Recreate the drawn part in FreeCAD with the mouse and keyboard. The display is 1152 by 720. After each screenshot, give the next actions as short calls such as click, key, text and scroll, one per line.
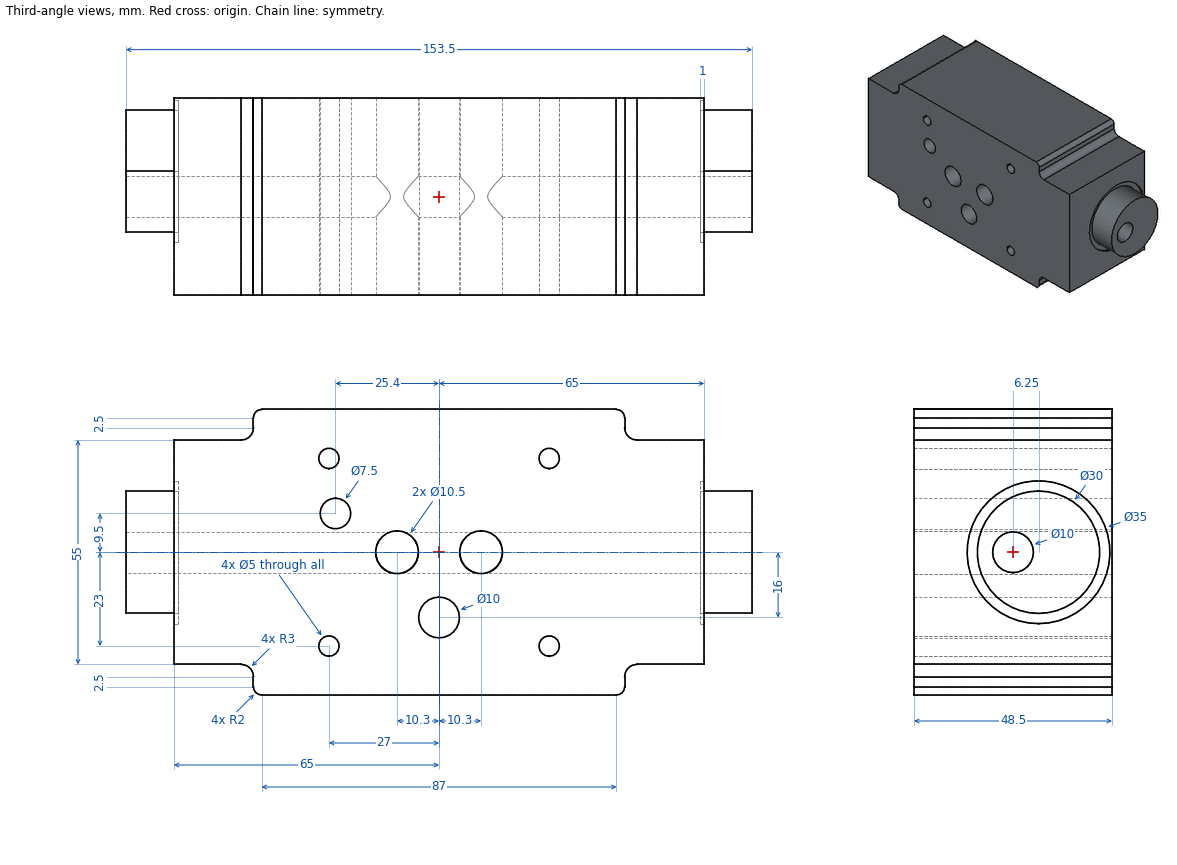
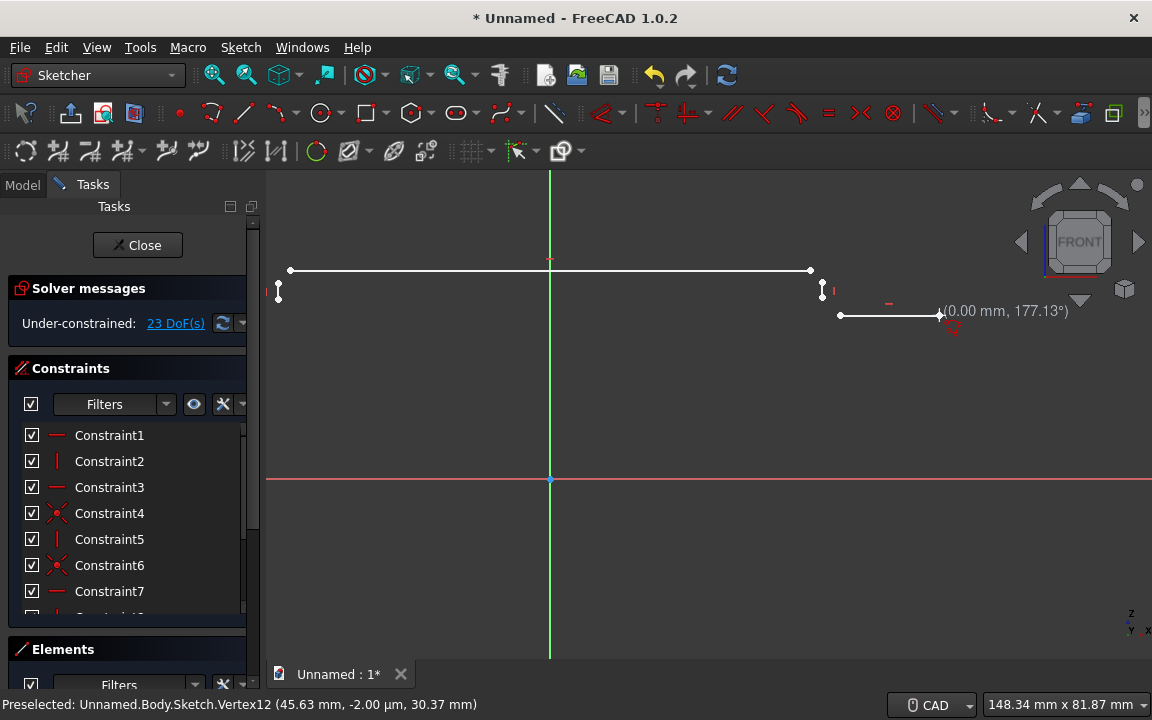
scroll(824, 283, down, 2)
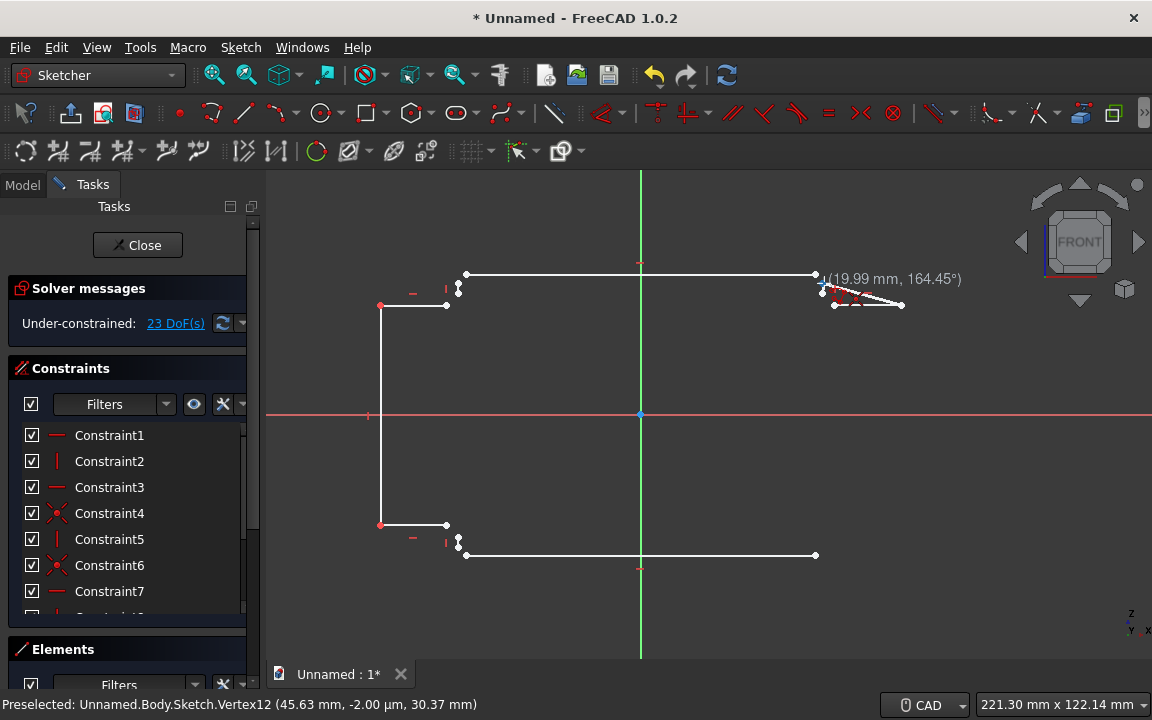
click(901, 525)
click(835, 525)
right_click(835, 525)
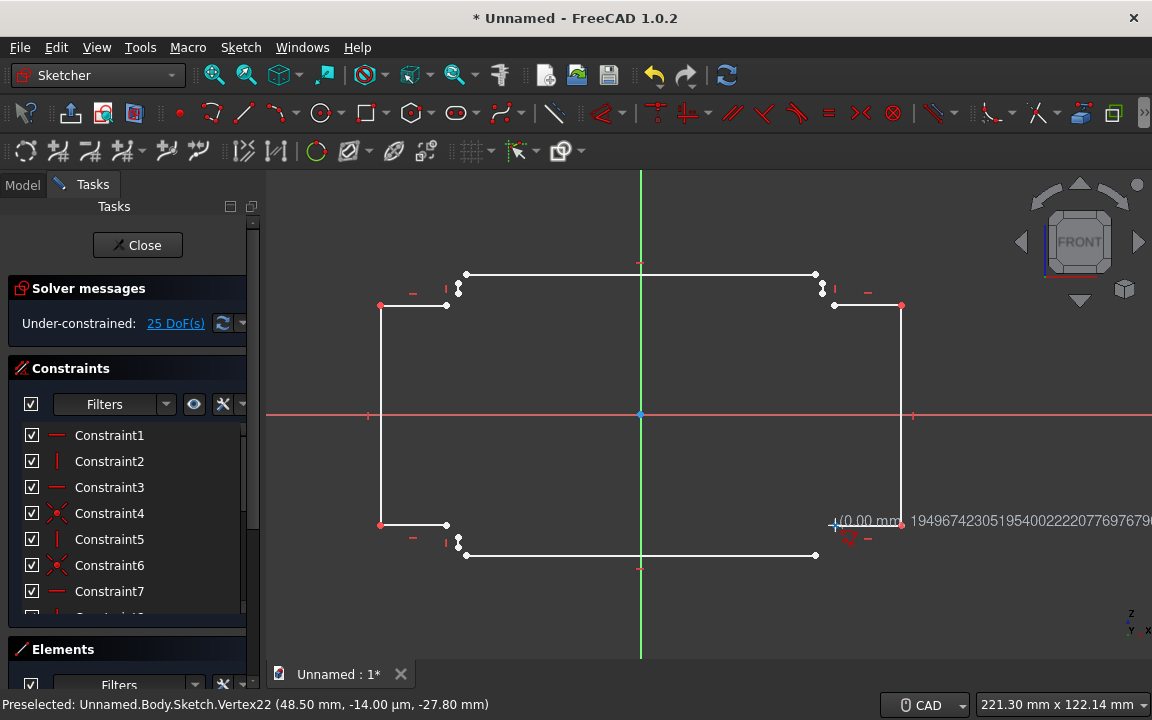
click(244, 114)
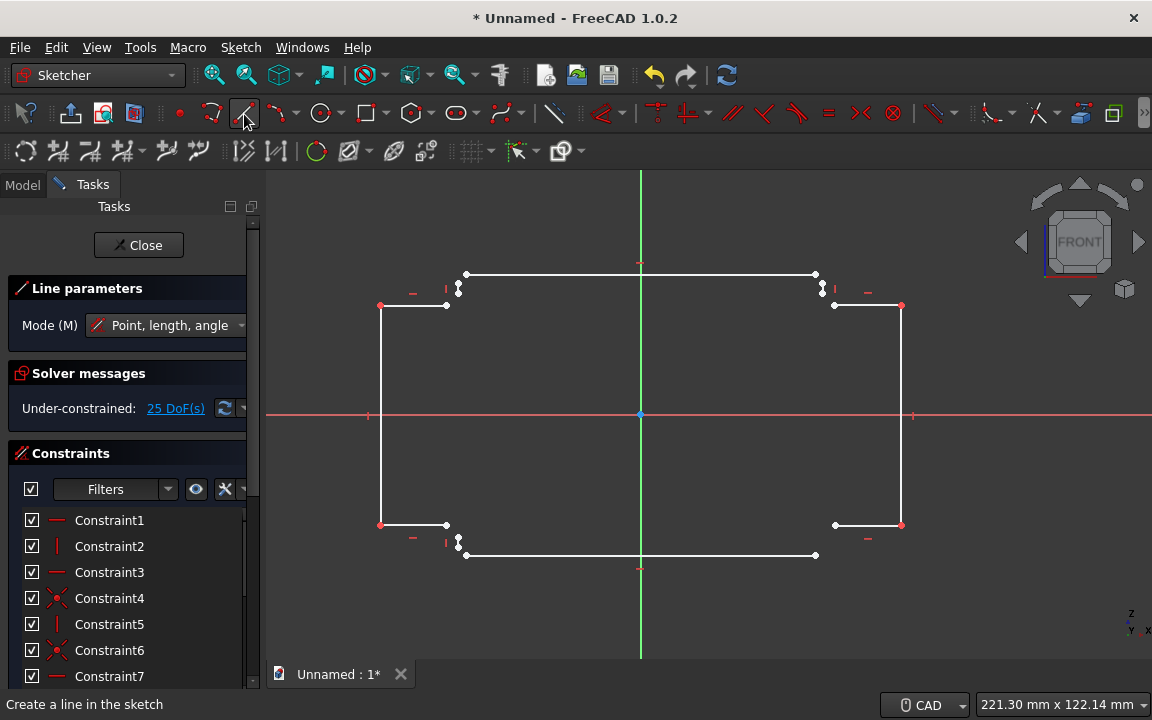
click(823, 537)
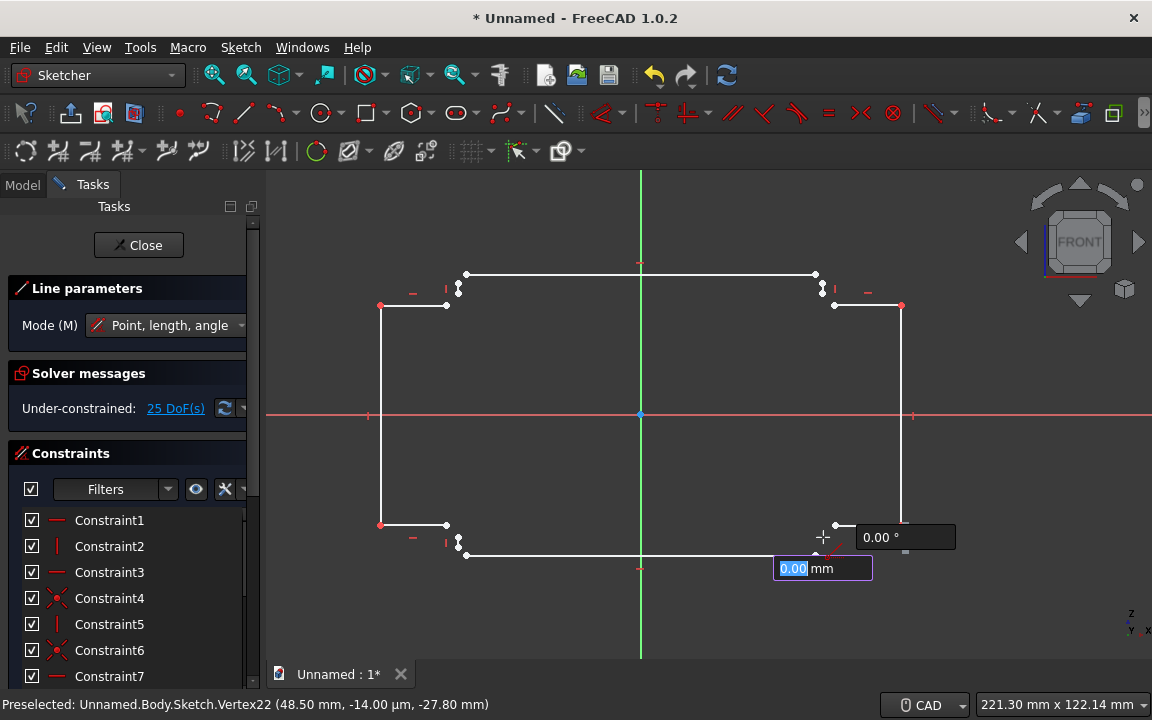
scroll(823, 547, up, 3)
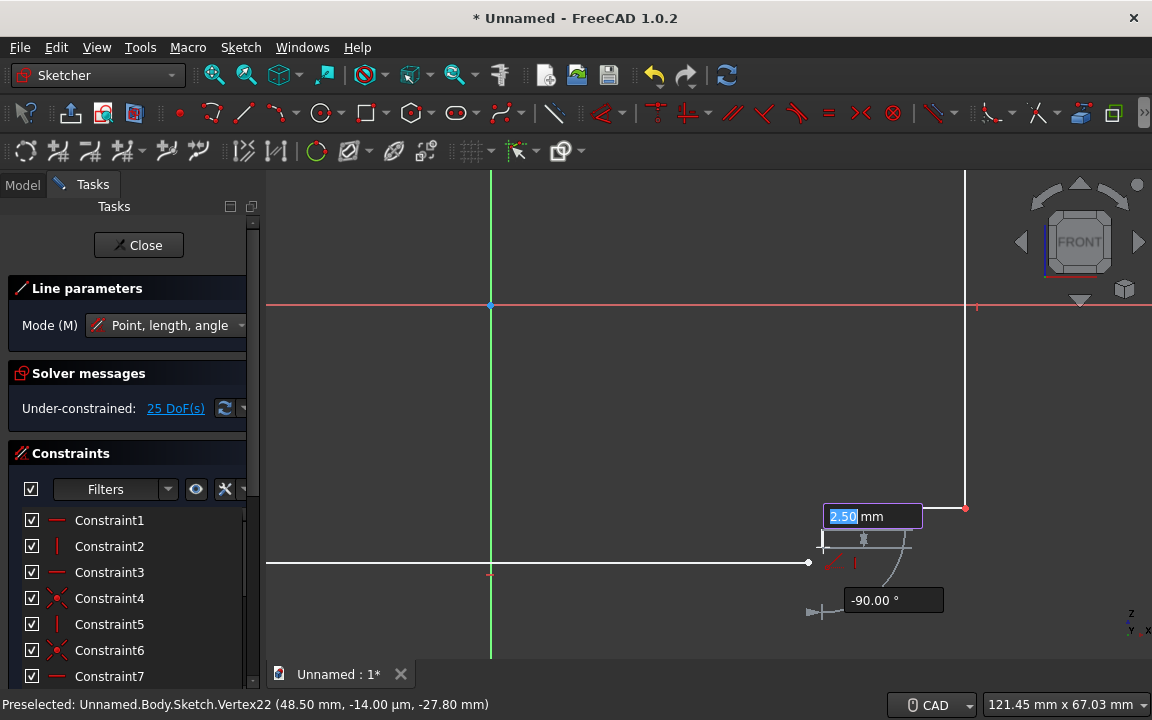
click(822, 546)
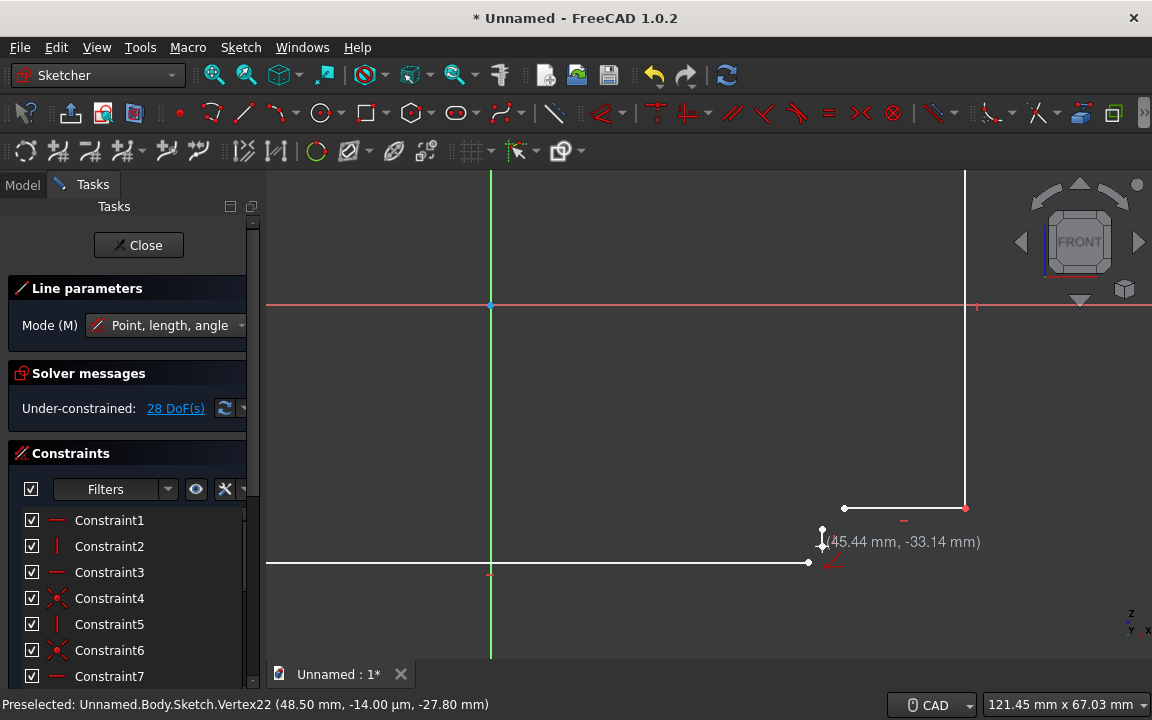
click(276, 114)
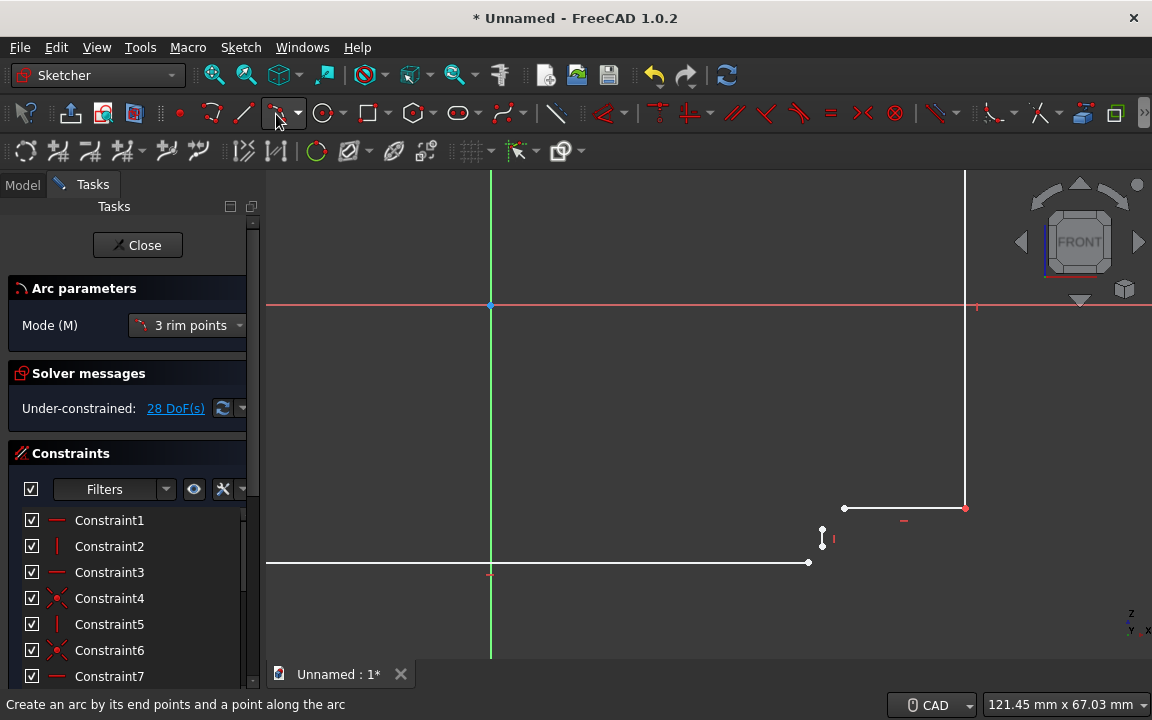
scroll(823, 547, down, 3)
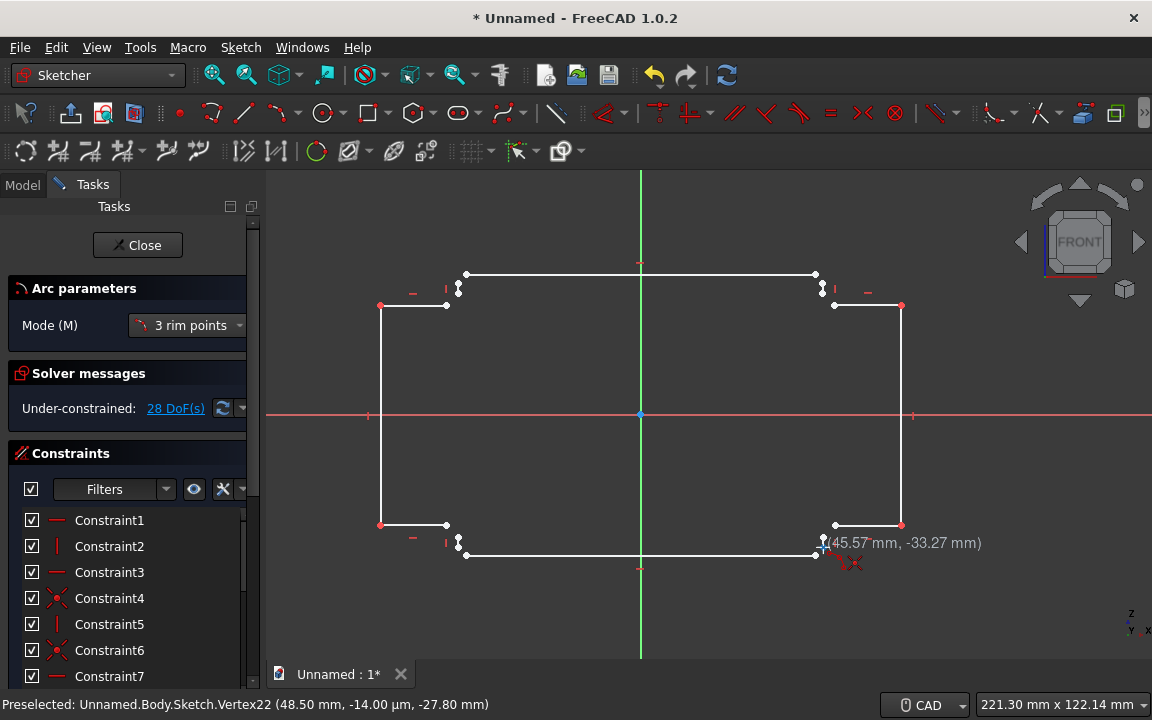
scroll(467, 555, up, 2)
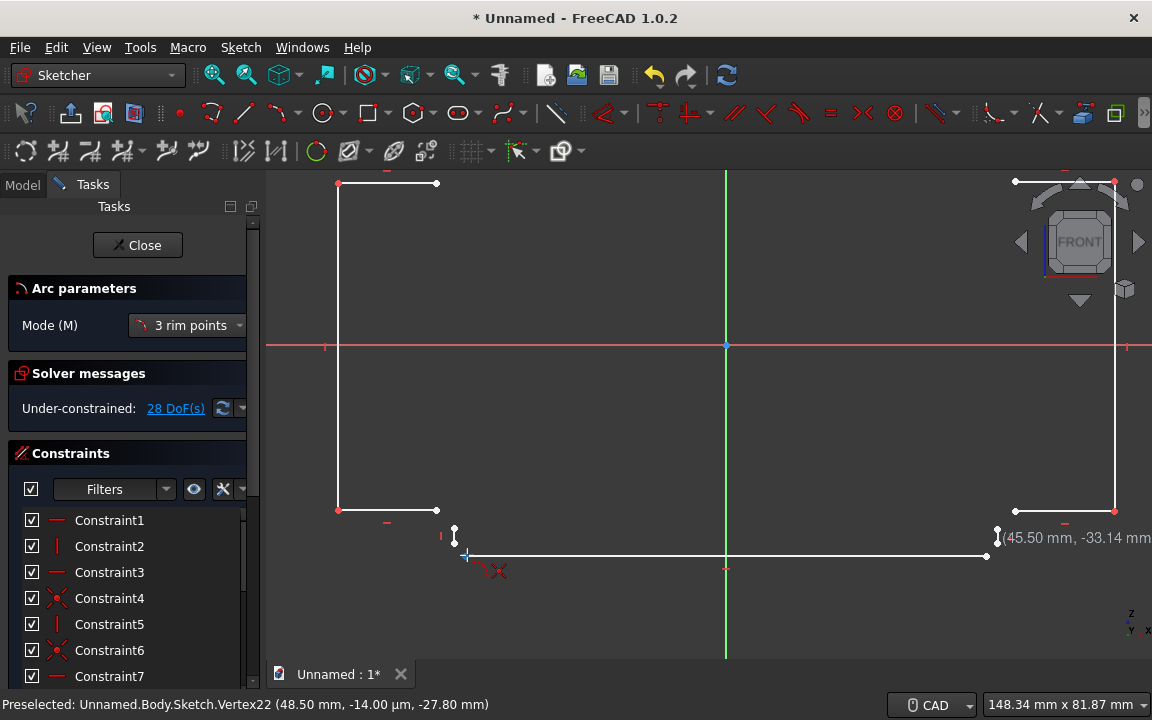
click(466, 556)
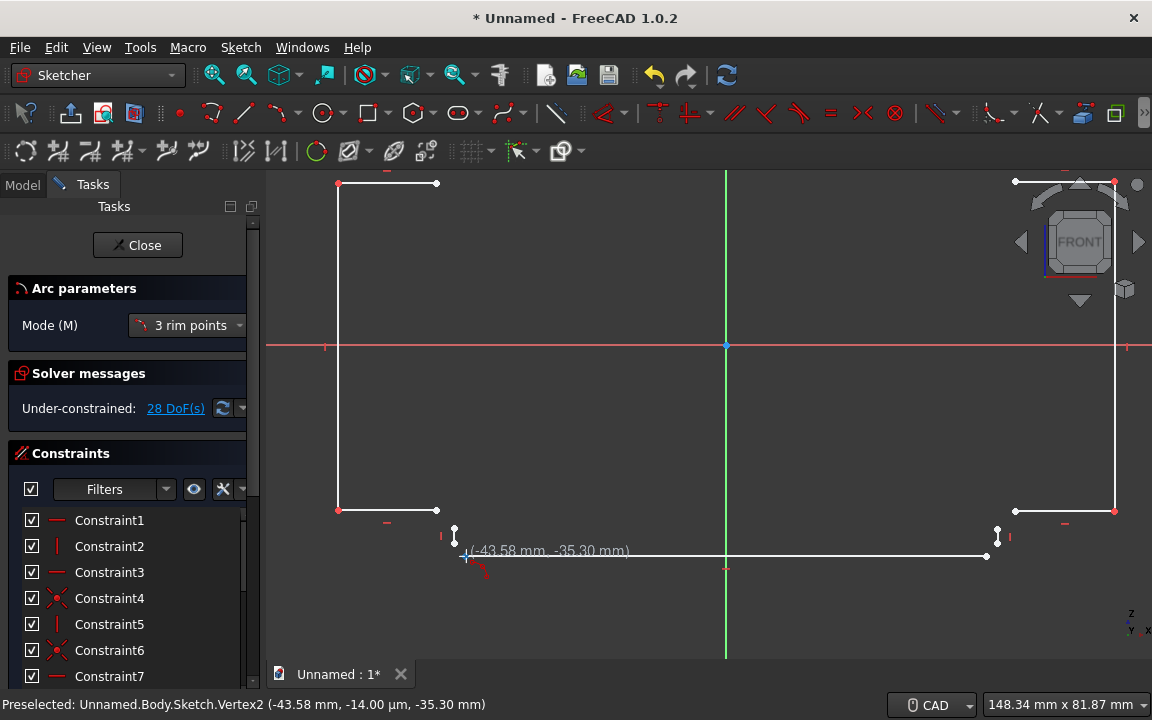
scroll(454, 542, up, 4)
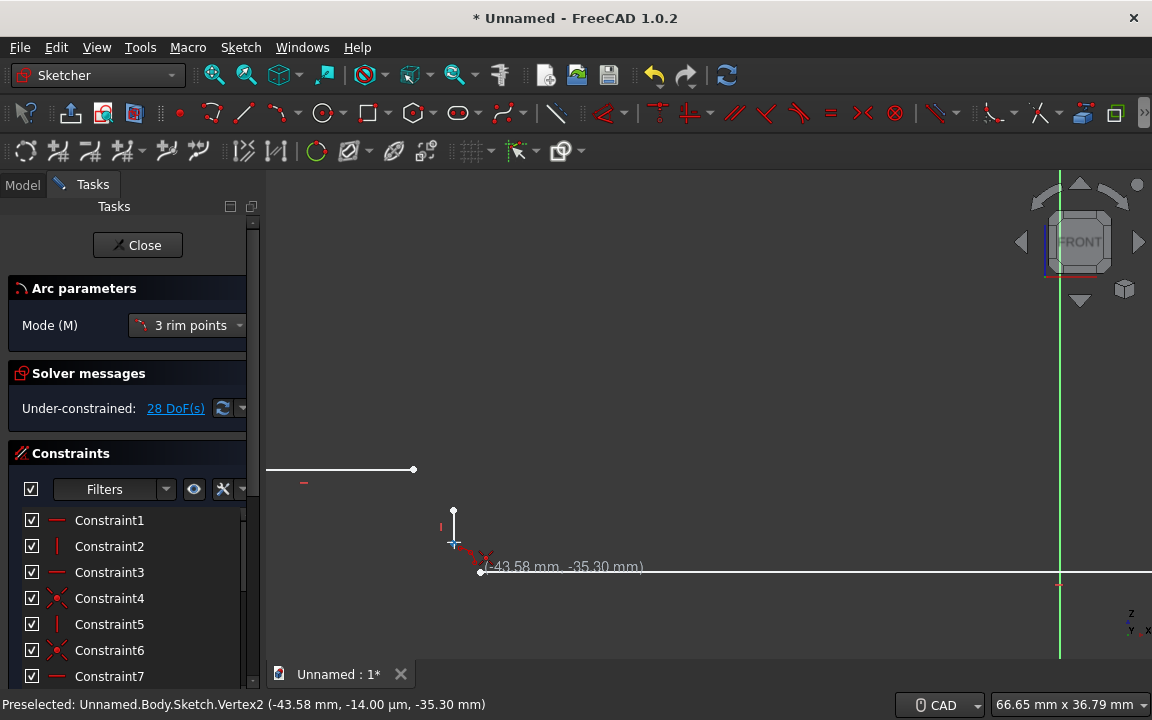
click(454, 543)